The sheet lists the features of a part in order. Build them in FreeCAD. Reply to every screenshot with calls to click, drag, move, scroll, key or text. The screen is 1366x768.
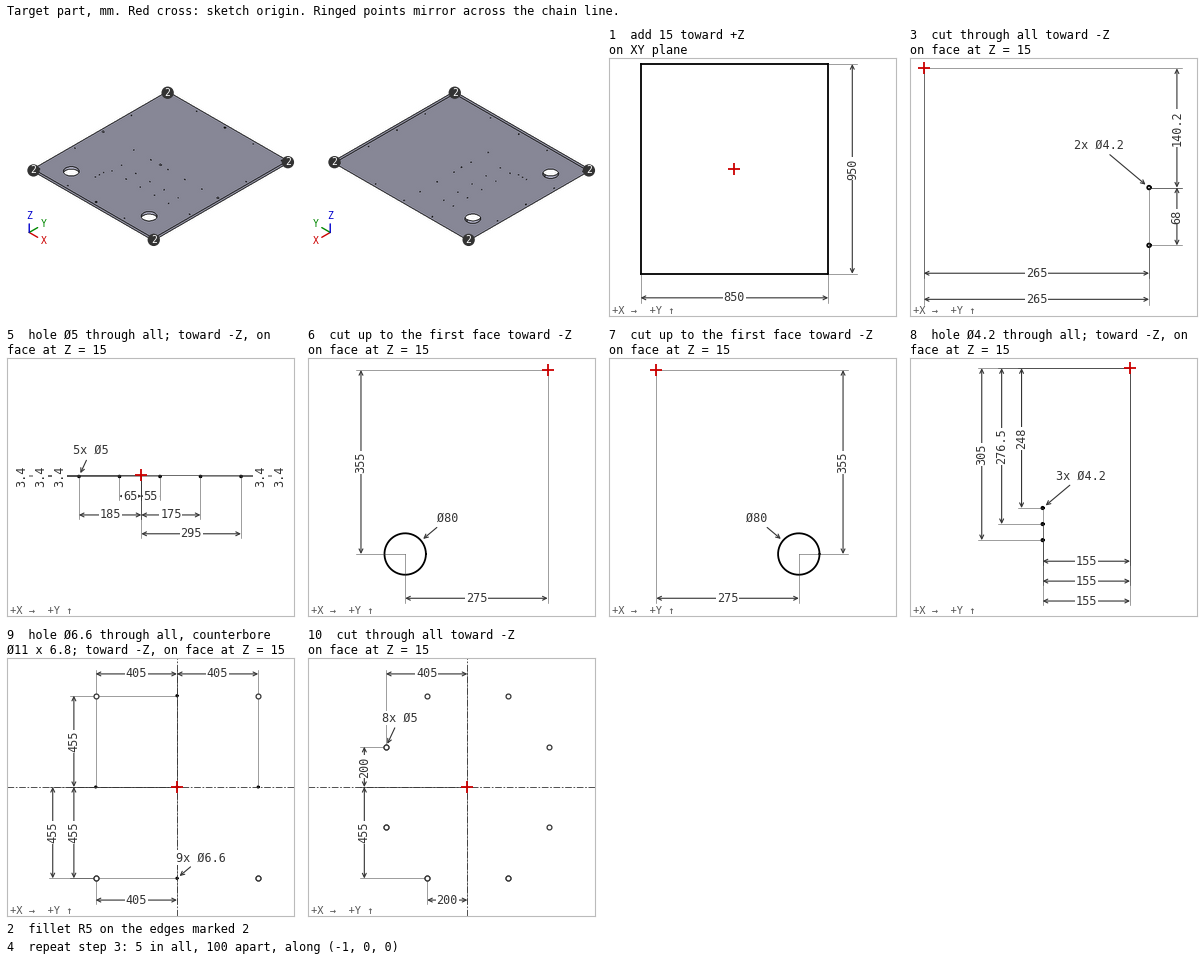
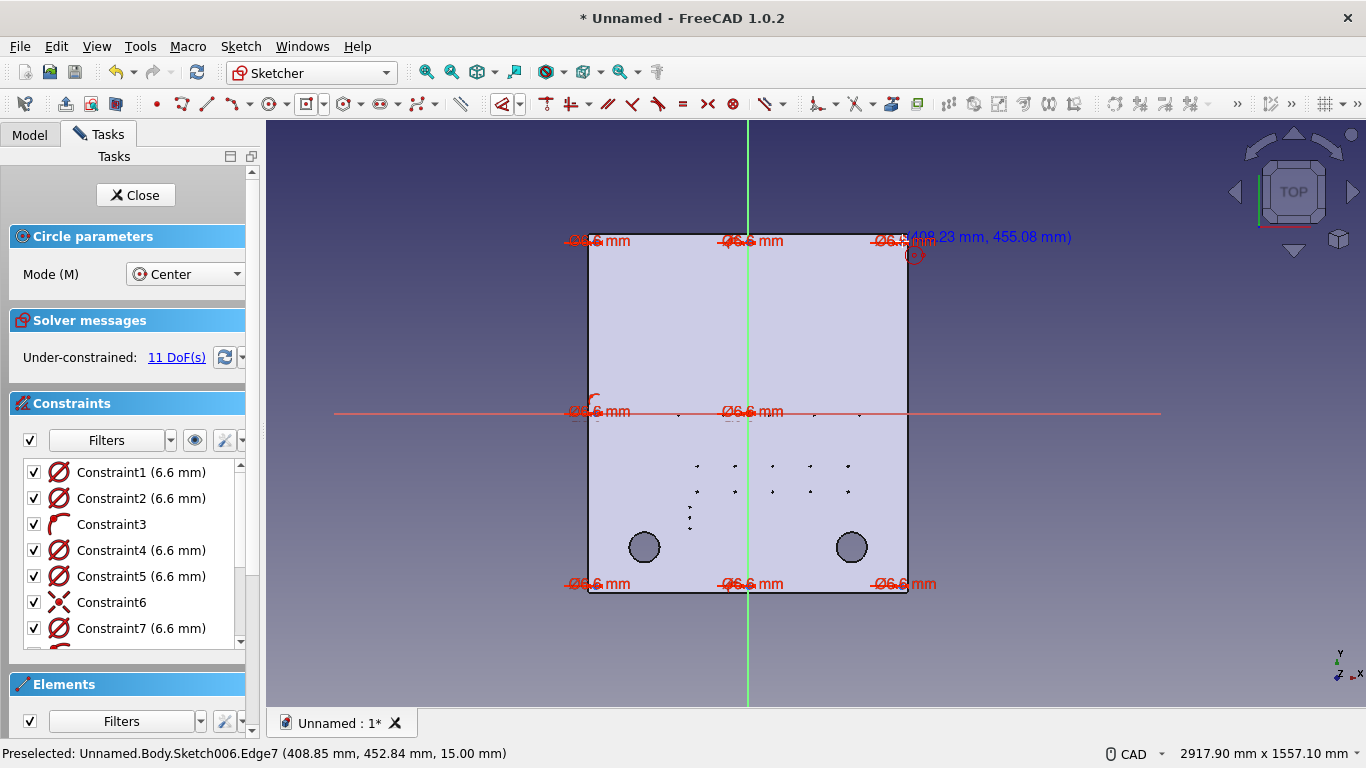
scroll(901, 414, up, 15)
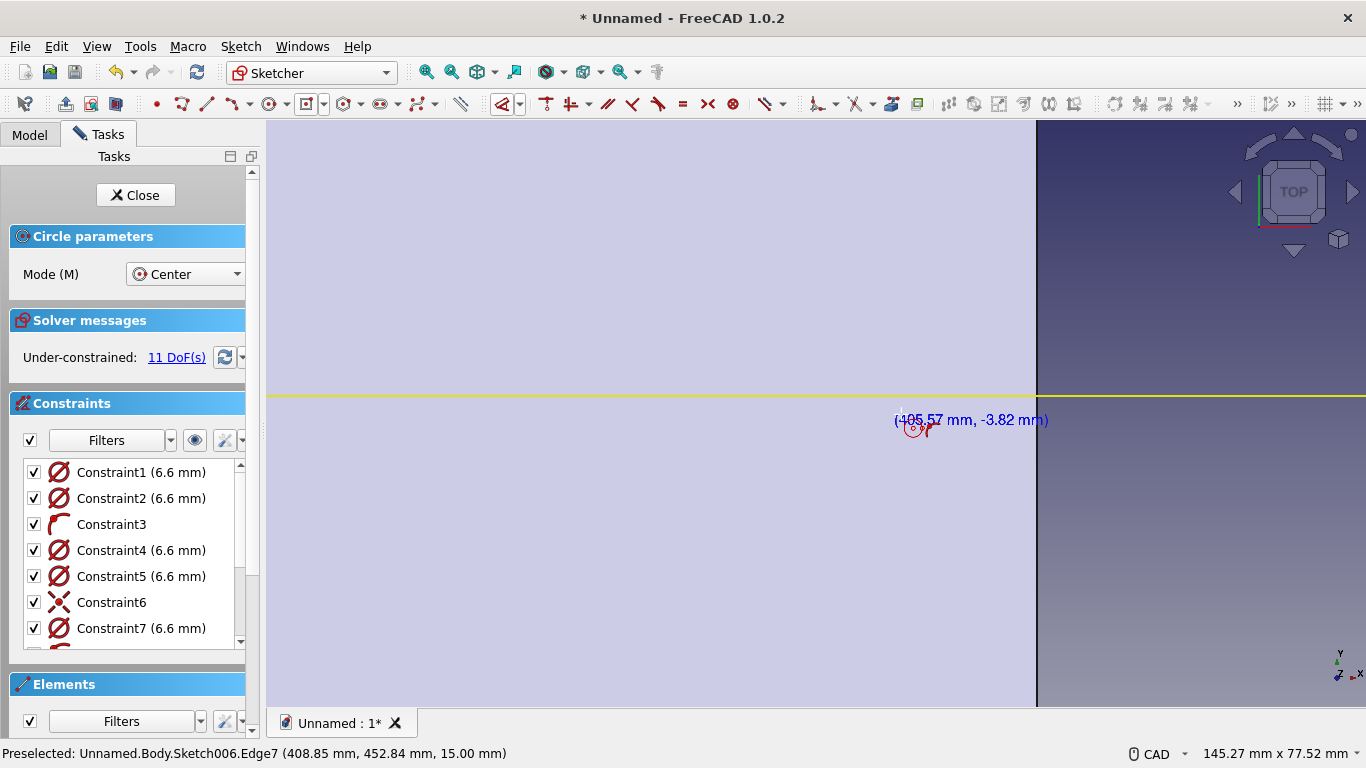
scroll(901, 414, down, 15)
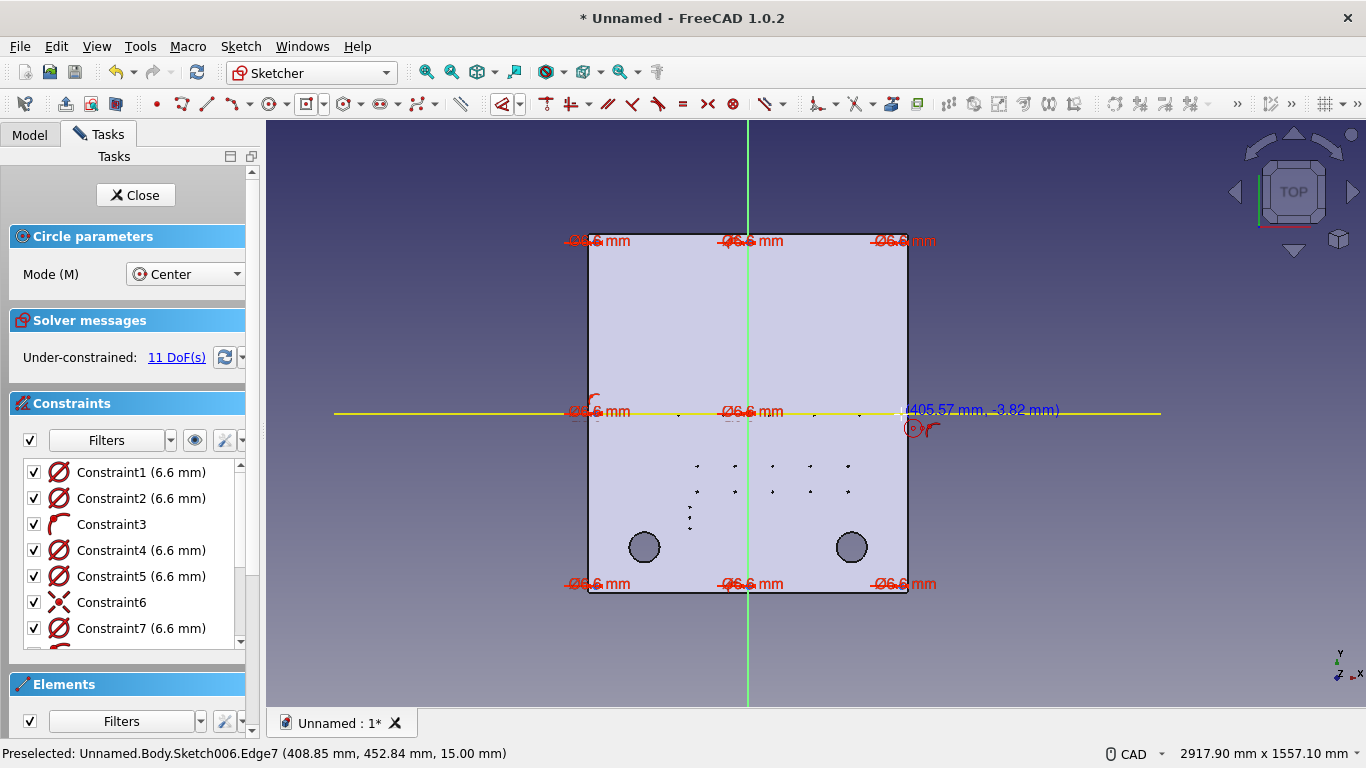
click(901, 414)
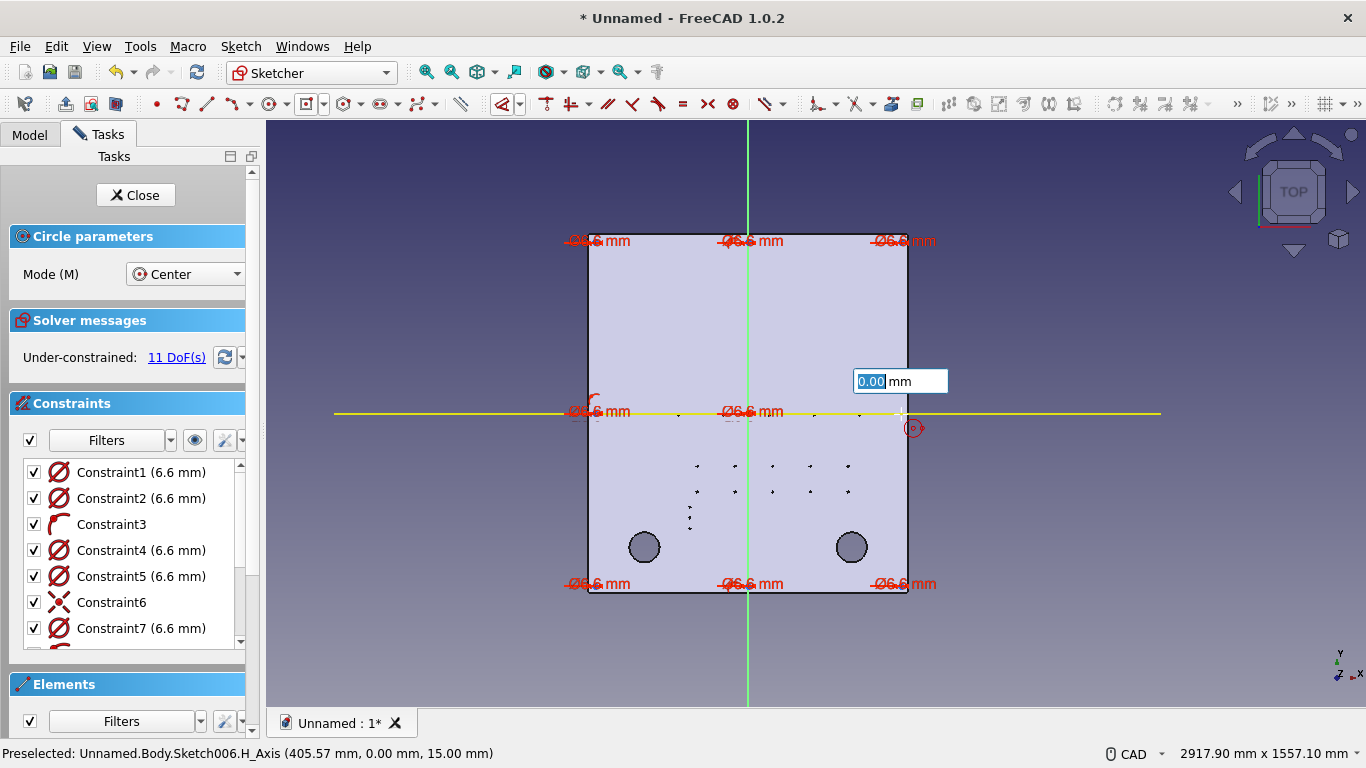
scroll(901, 412, up, 14)
move(896, 411)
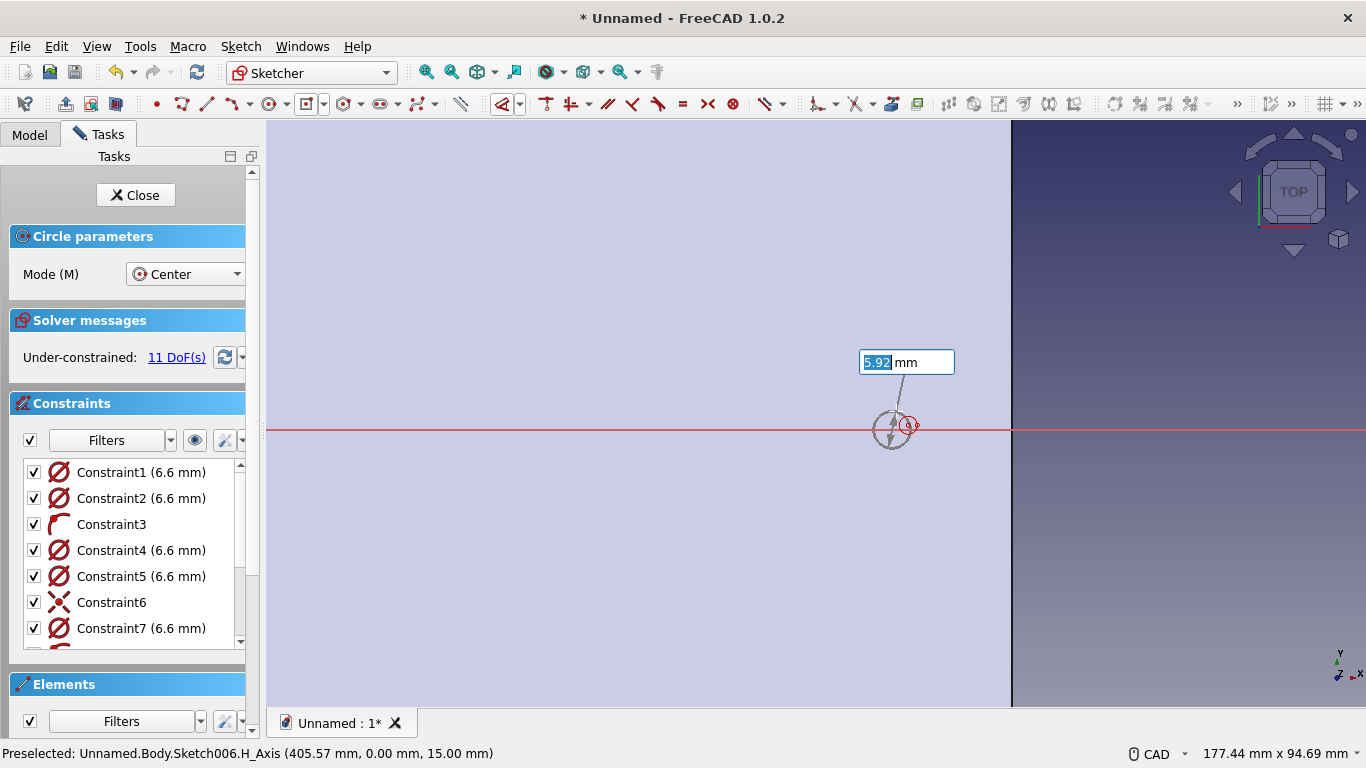
text(6.6)
key(Return)
key(Escape)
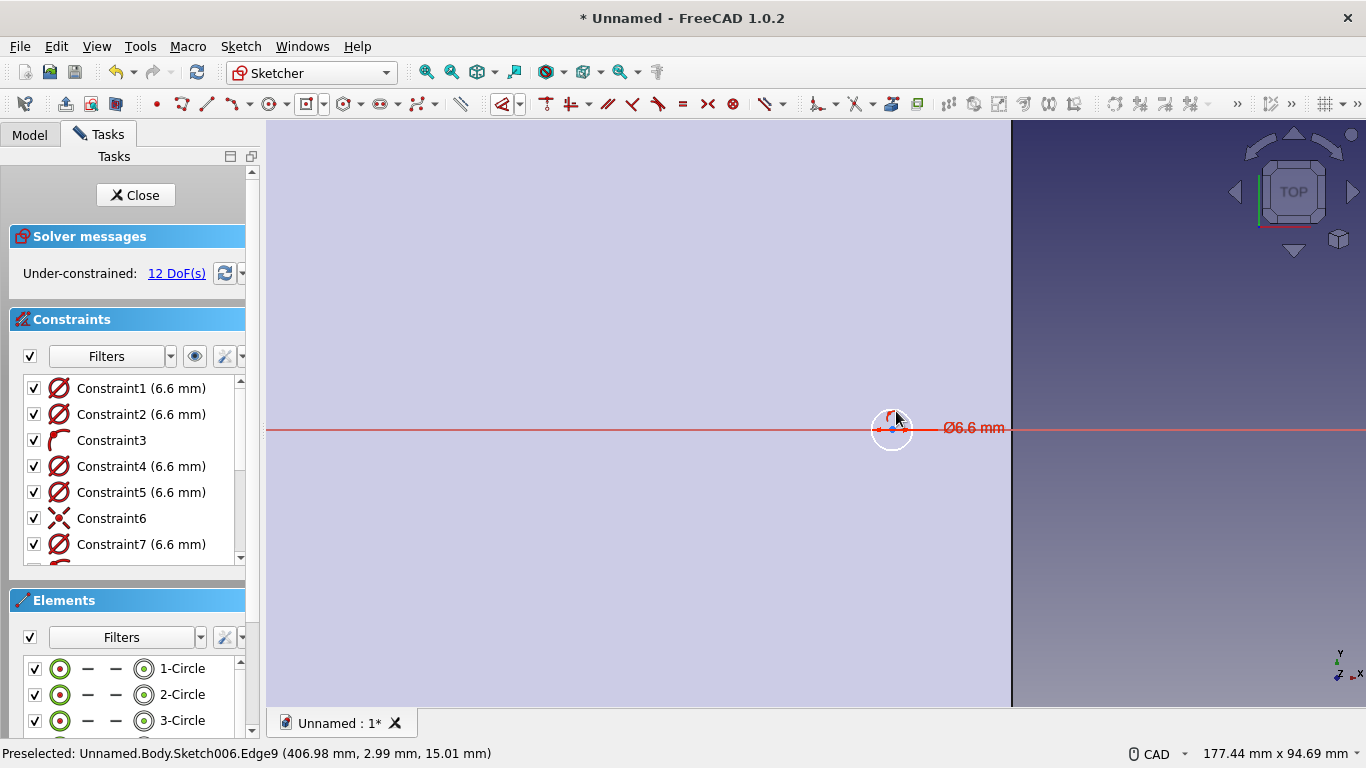
scroll(901, 412, down, 14)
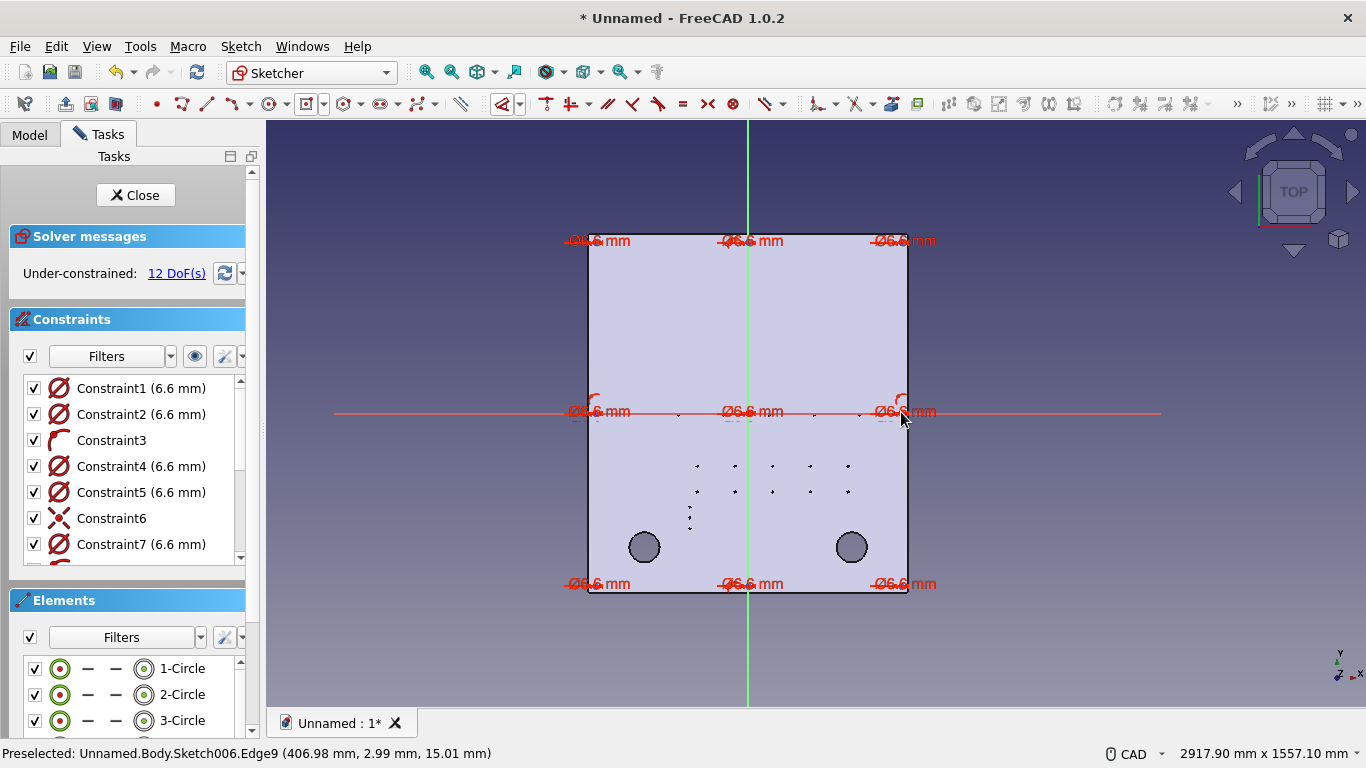
click(595, 586)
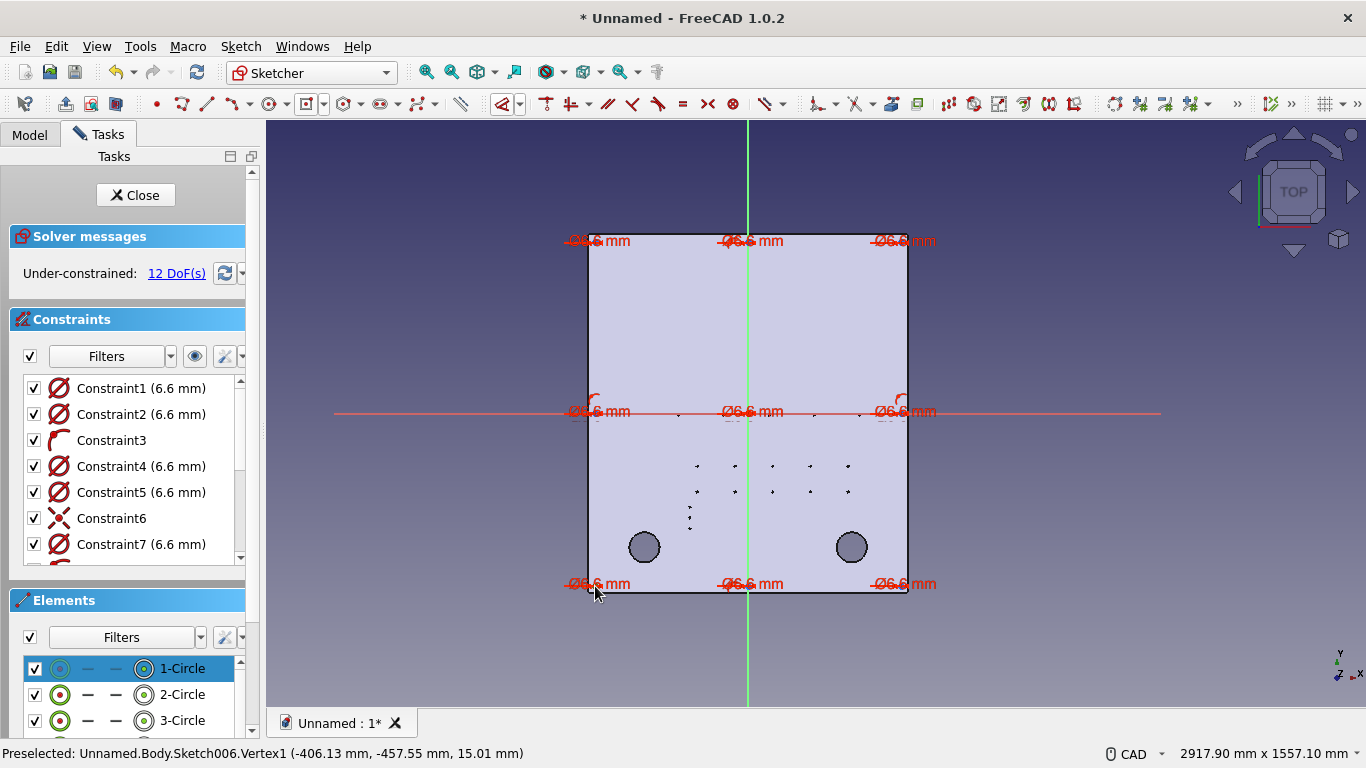
click(901, 586)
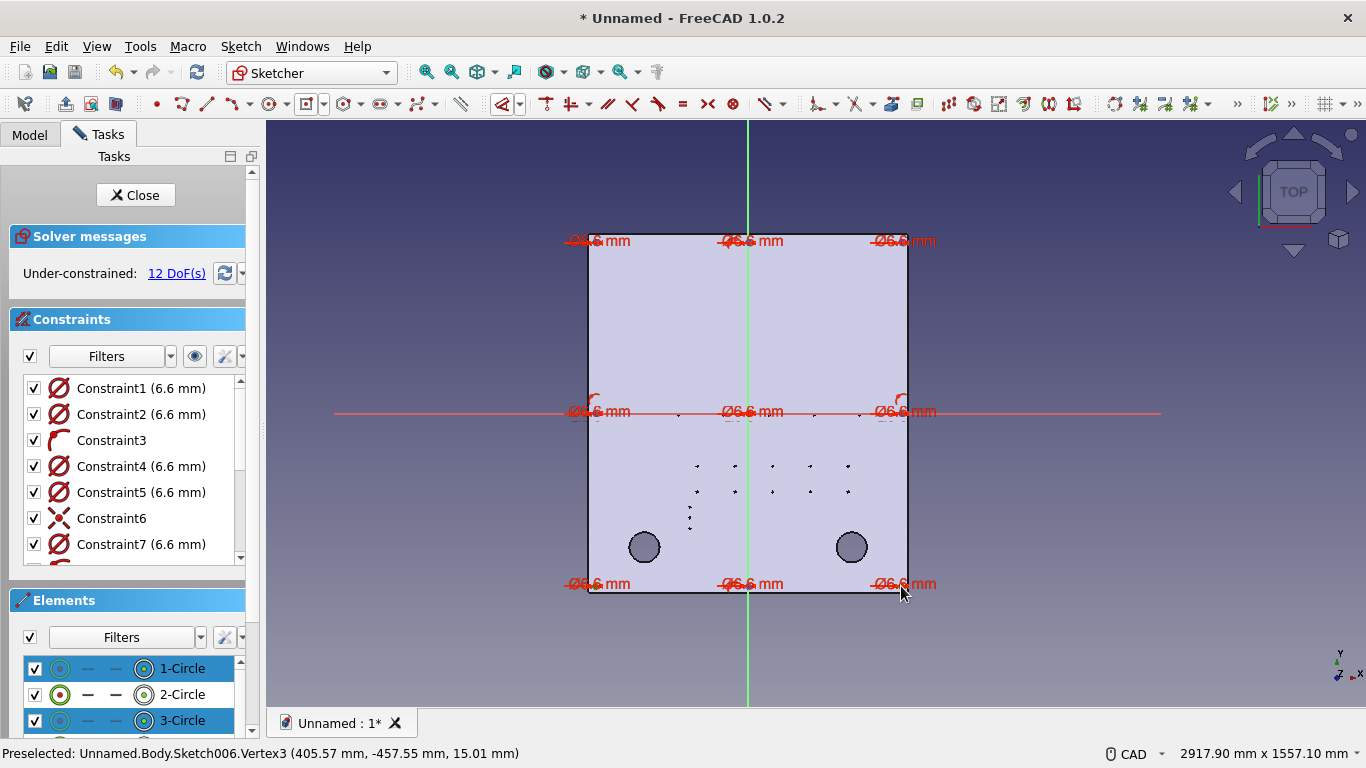
click(748, 641)